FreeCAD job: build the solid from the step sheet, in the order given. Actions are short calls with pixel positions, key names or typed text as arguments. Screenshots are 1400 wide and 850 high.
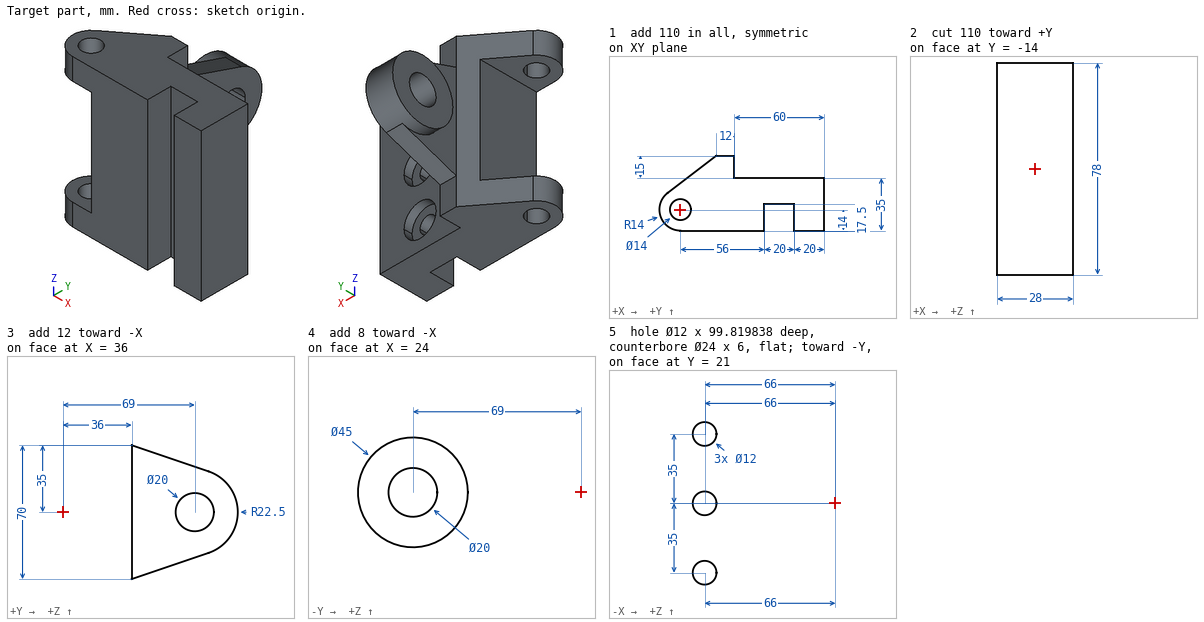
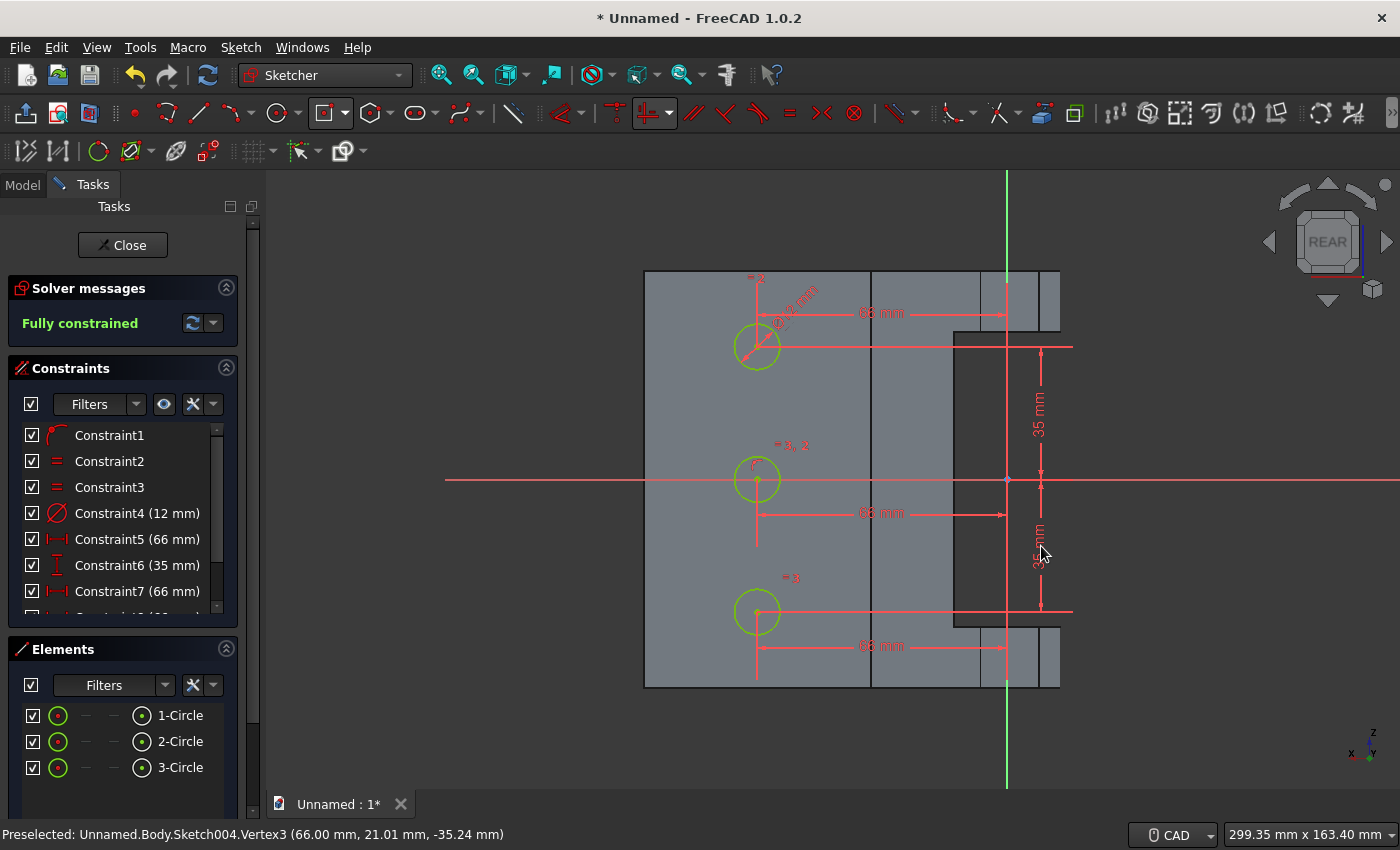
click(123, 245)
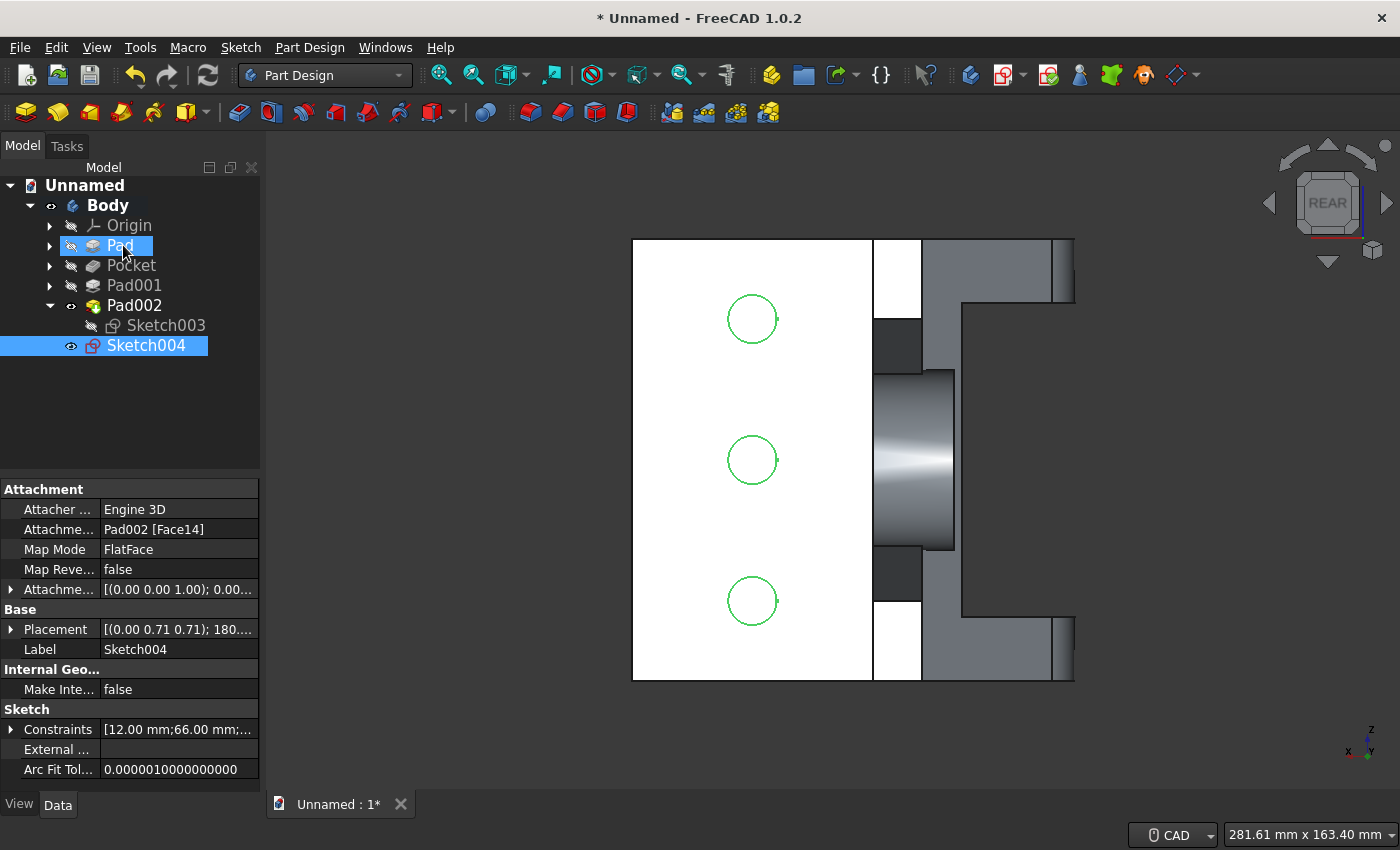
click(272, 112)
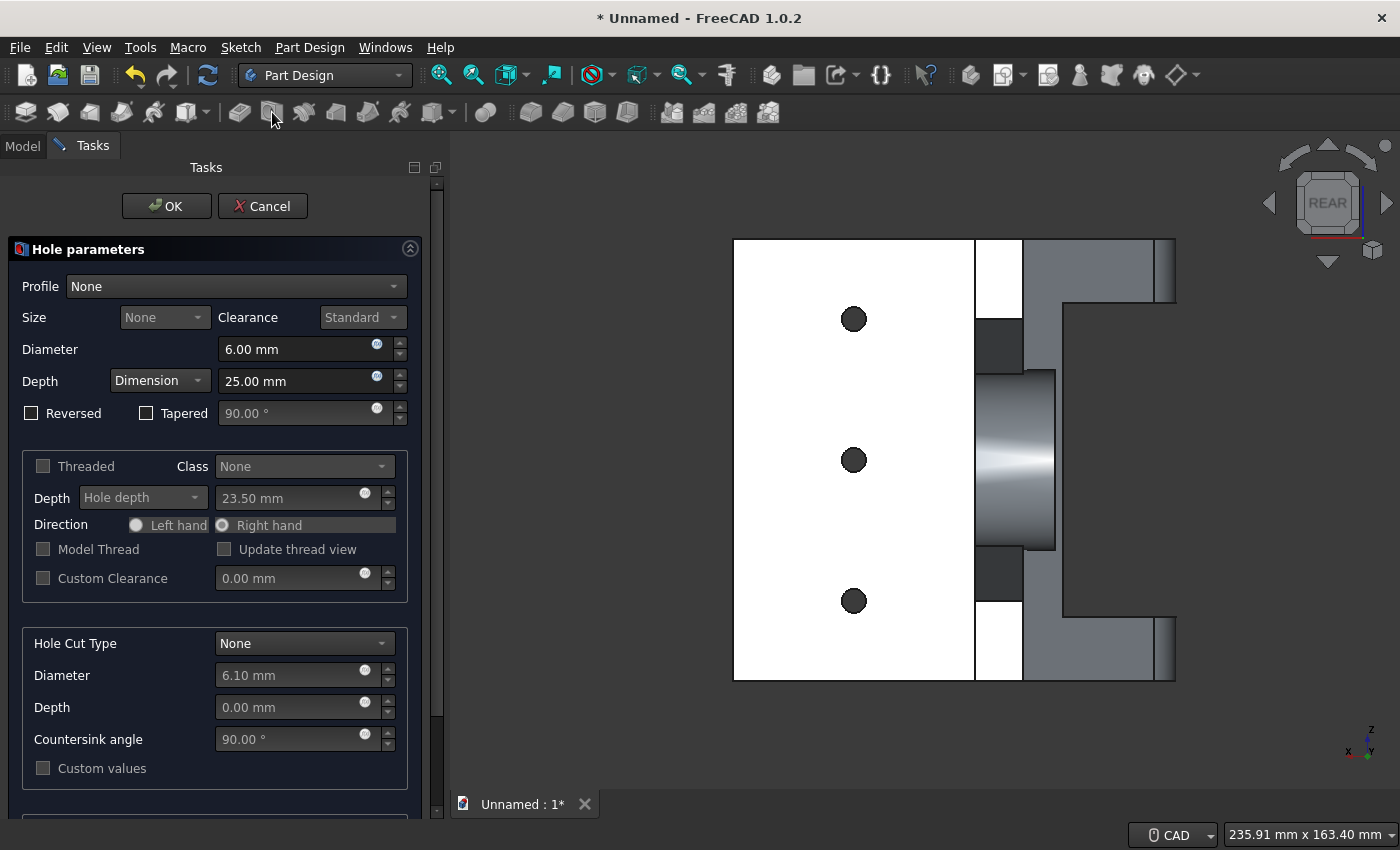
triple_click(305, 349)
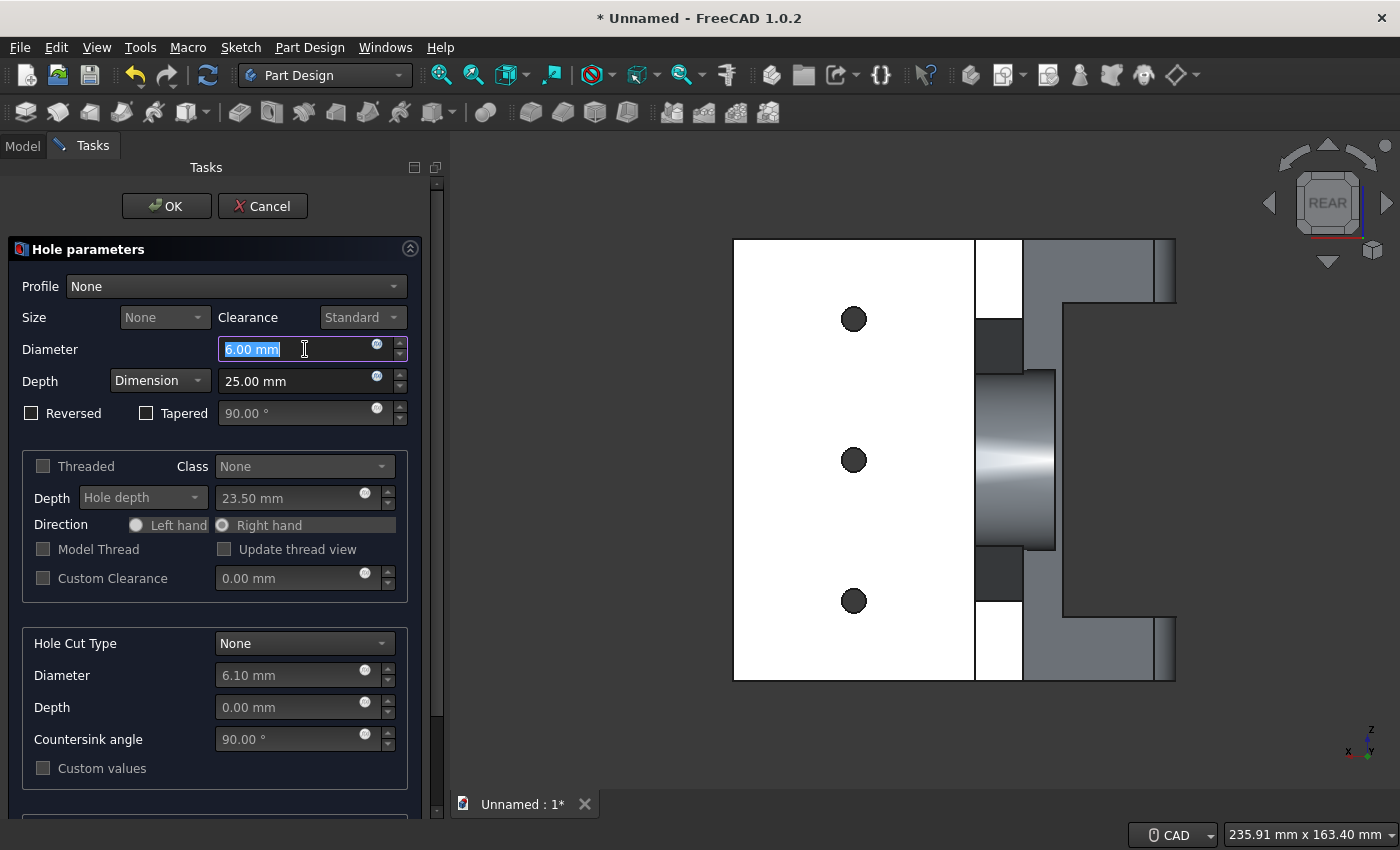
text(12)
key(Tab)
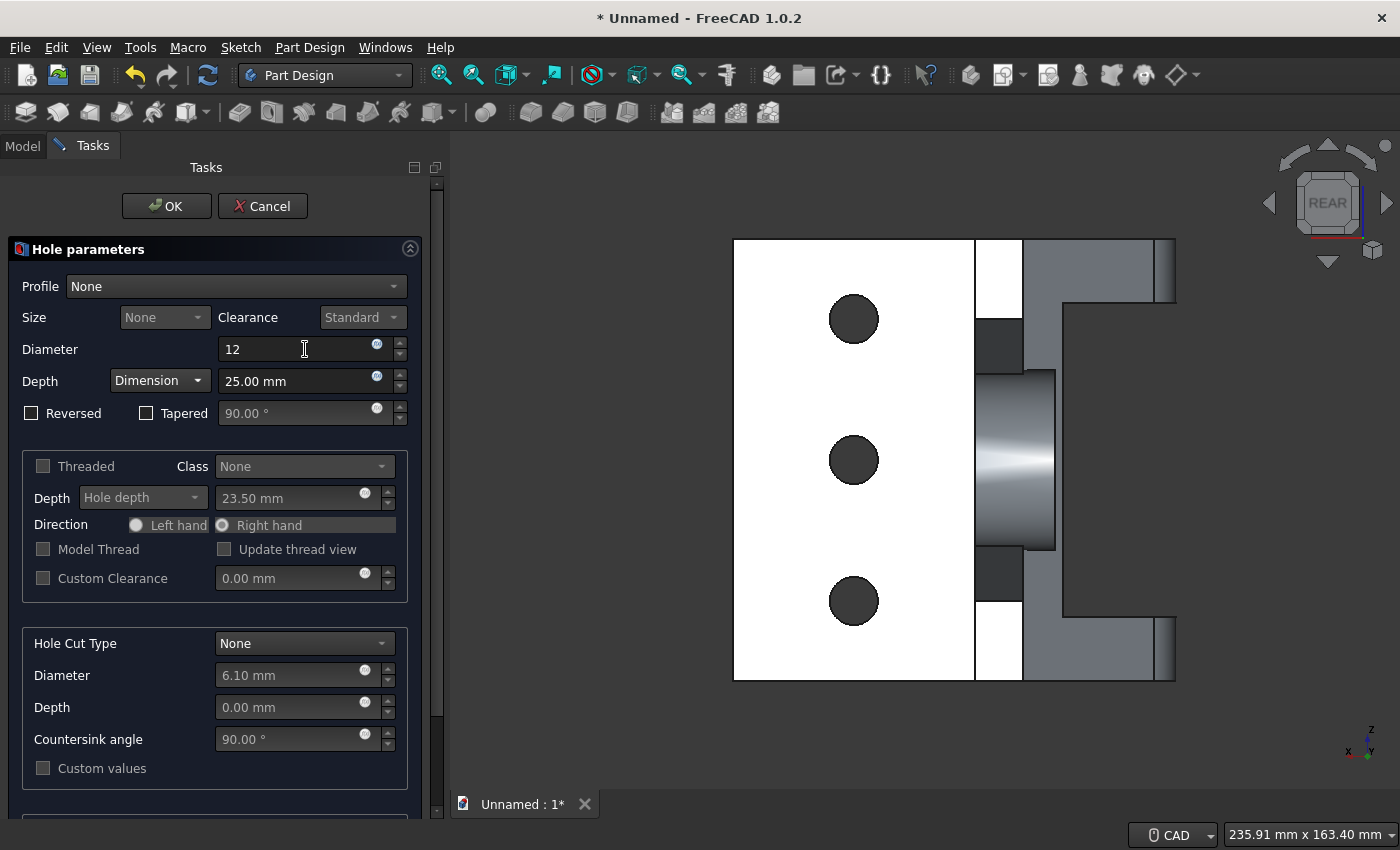
triple_click(305, 381)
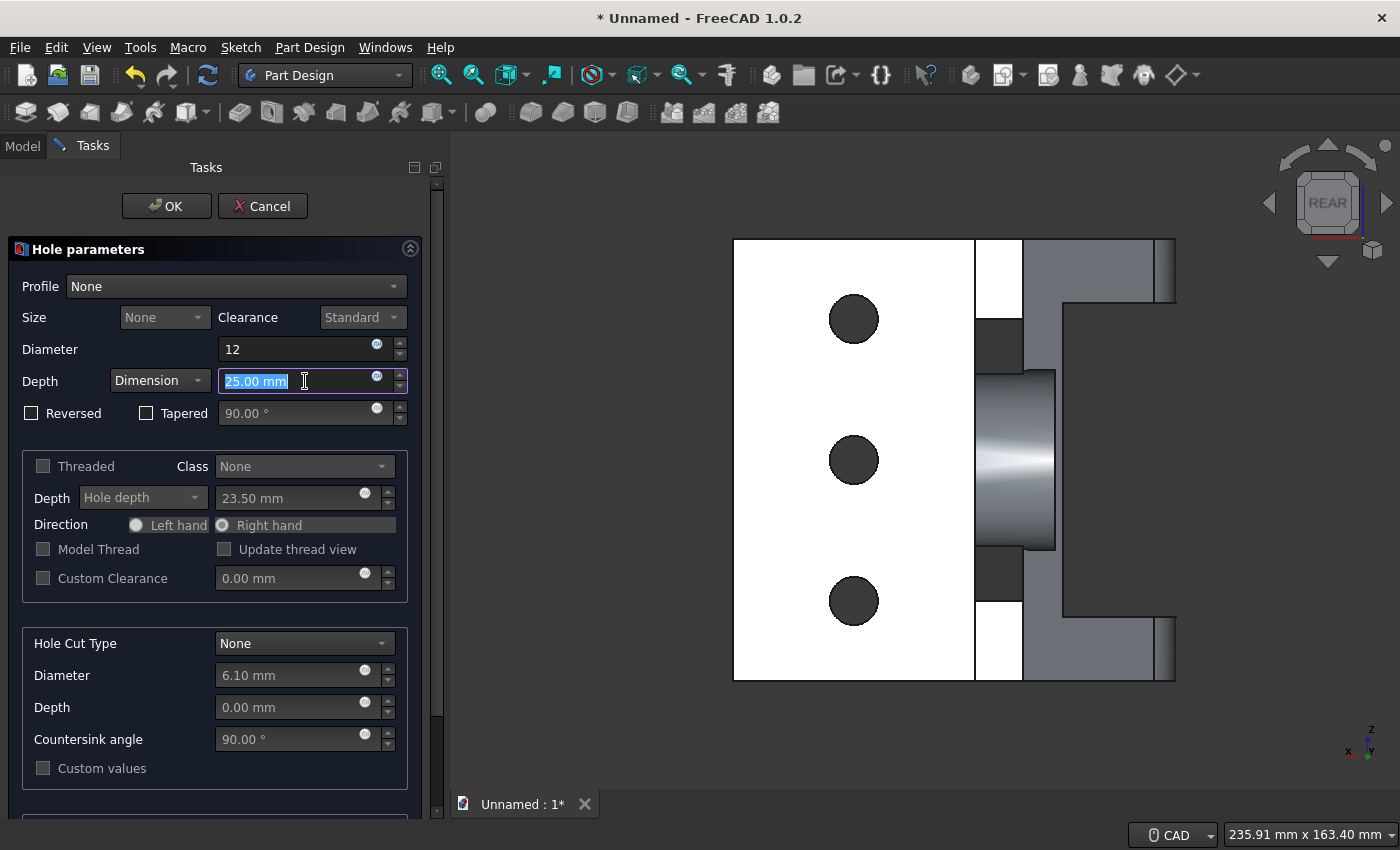
text(99.819838)
key(Tab)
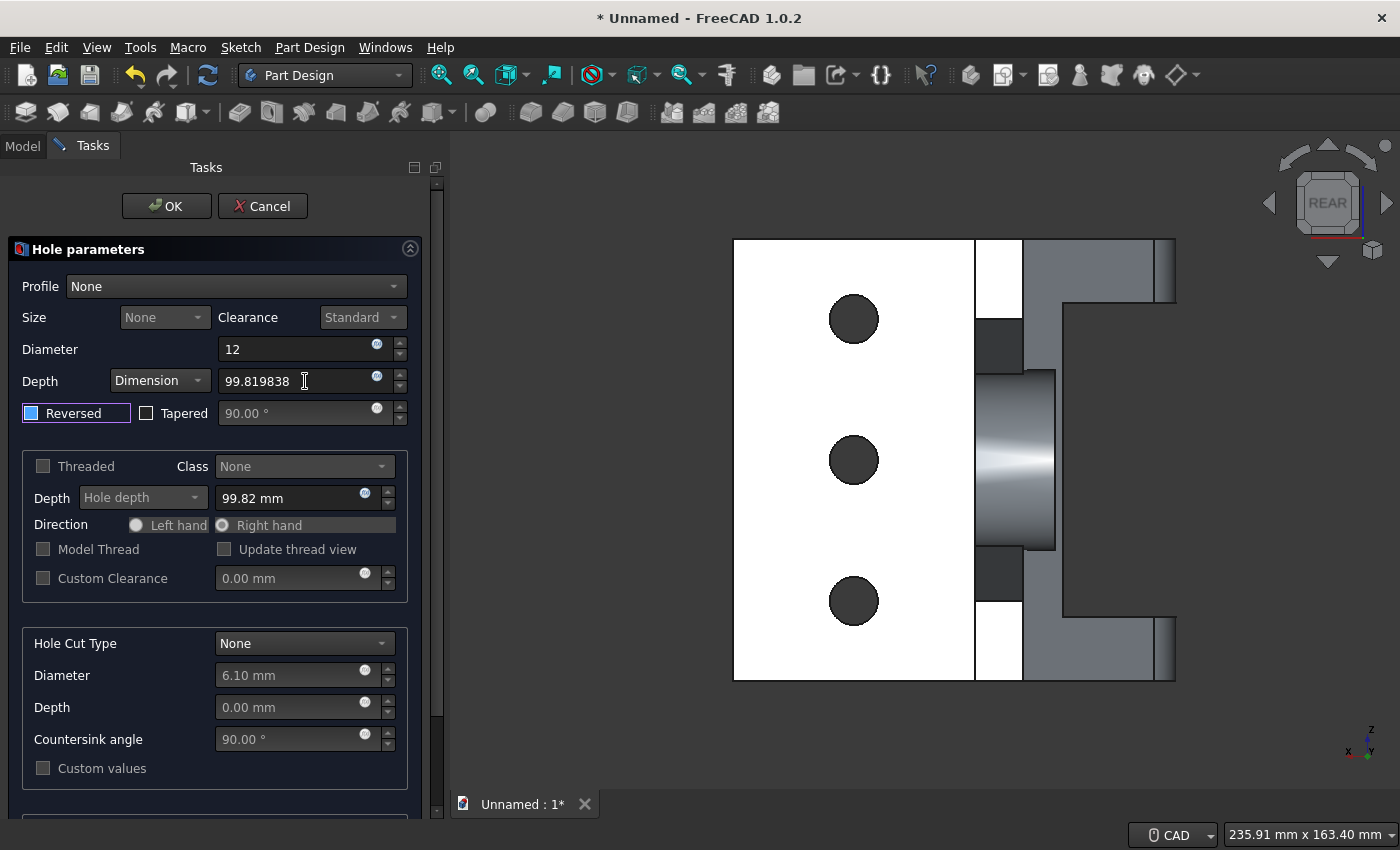
click(306, 644)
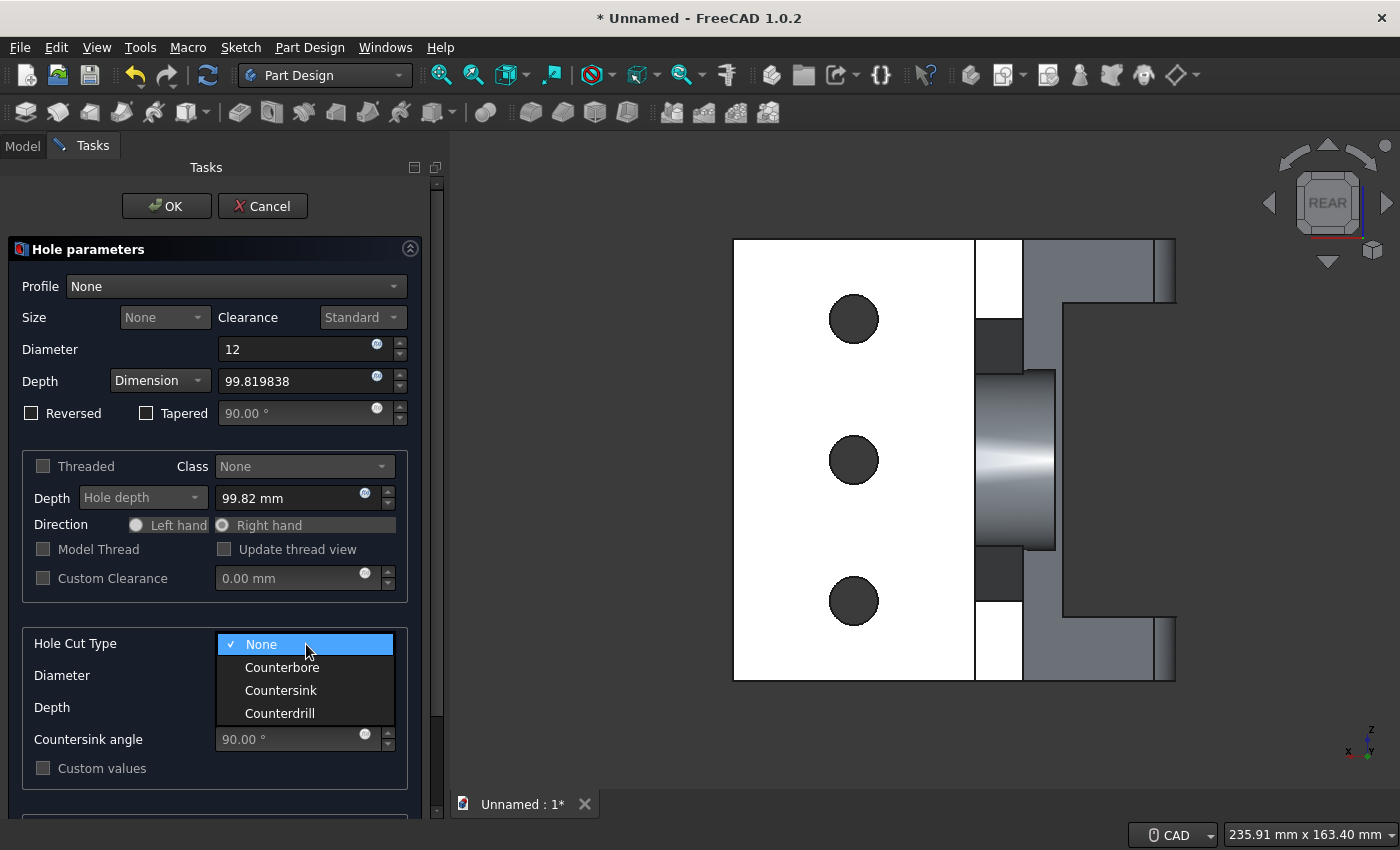
click(304, 668)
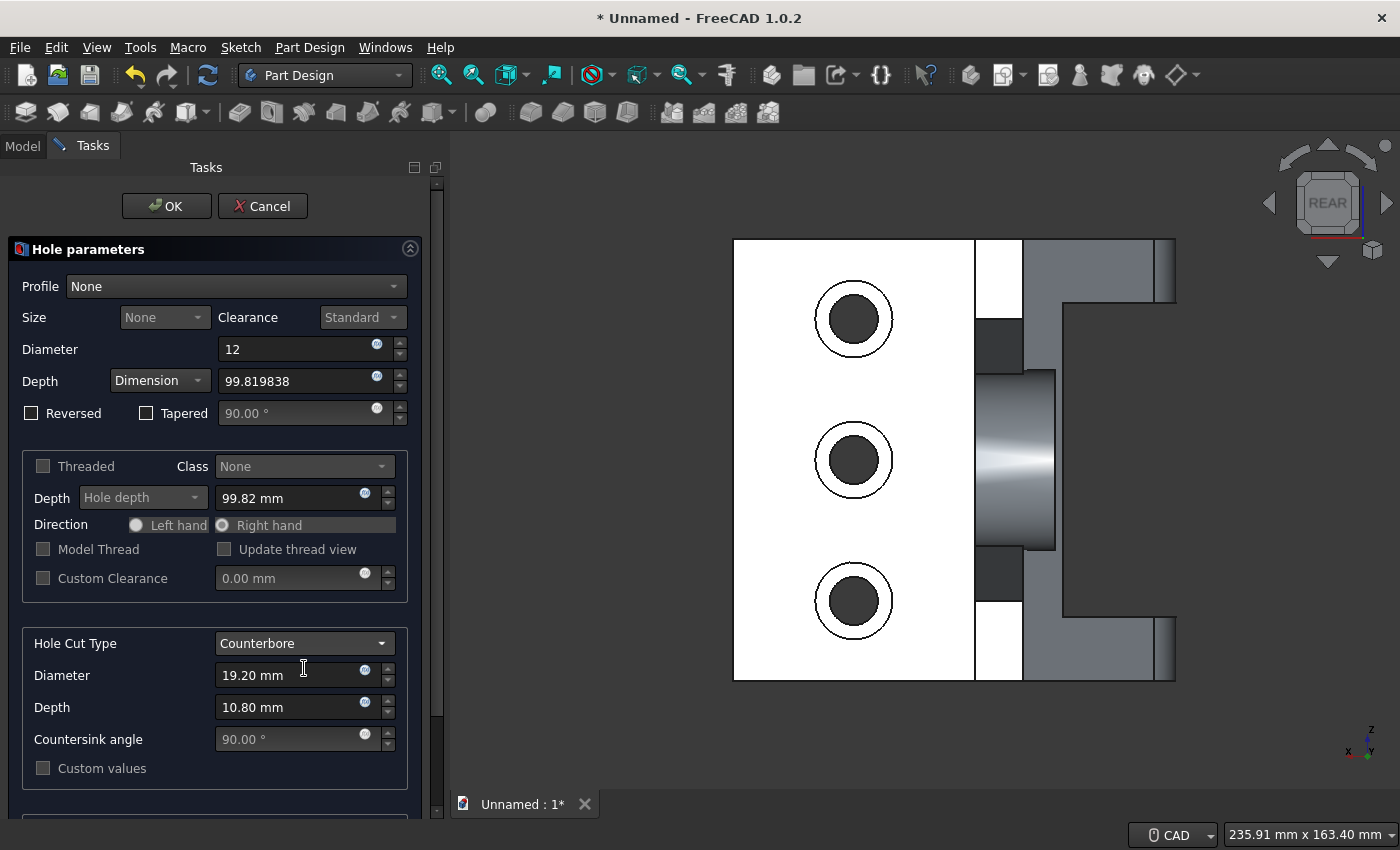
triple_click(298, 675)